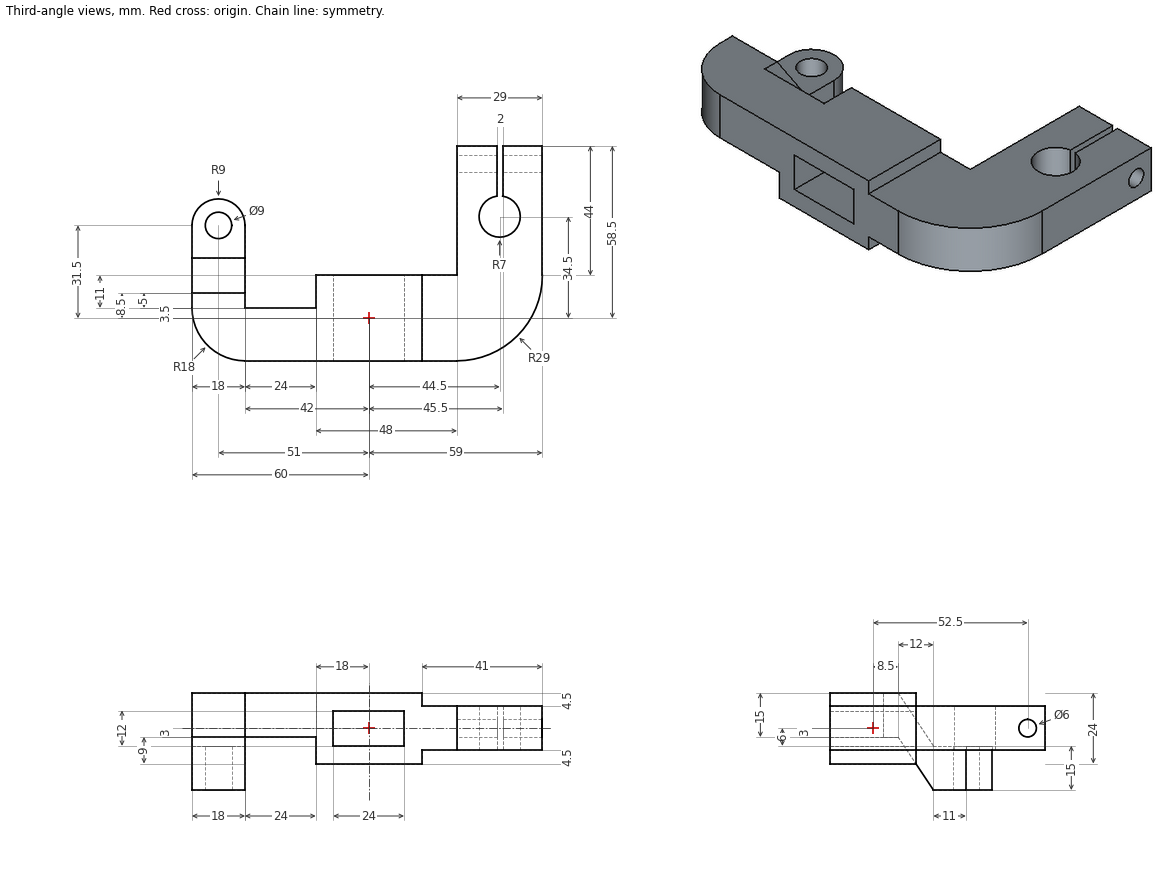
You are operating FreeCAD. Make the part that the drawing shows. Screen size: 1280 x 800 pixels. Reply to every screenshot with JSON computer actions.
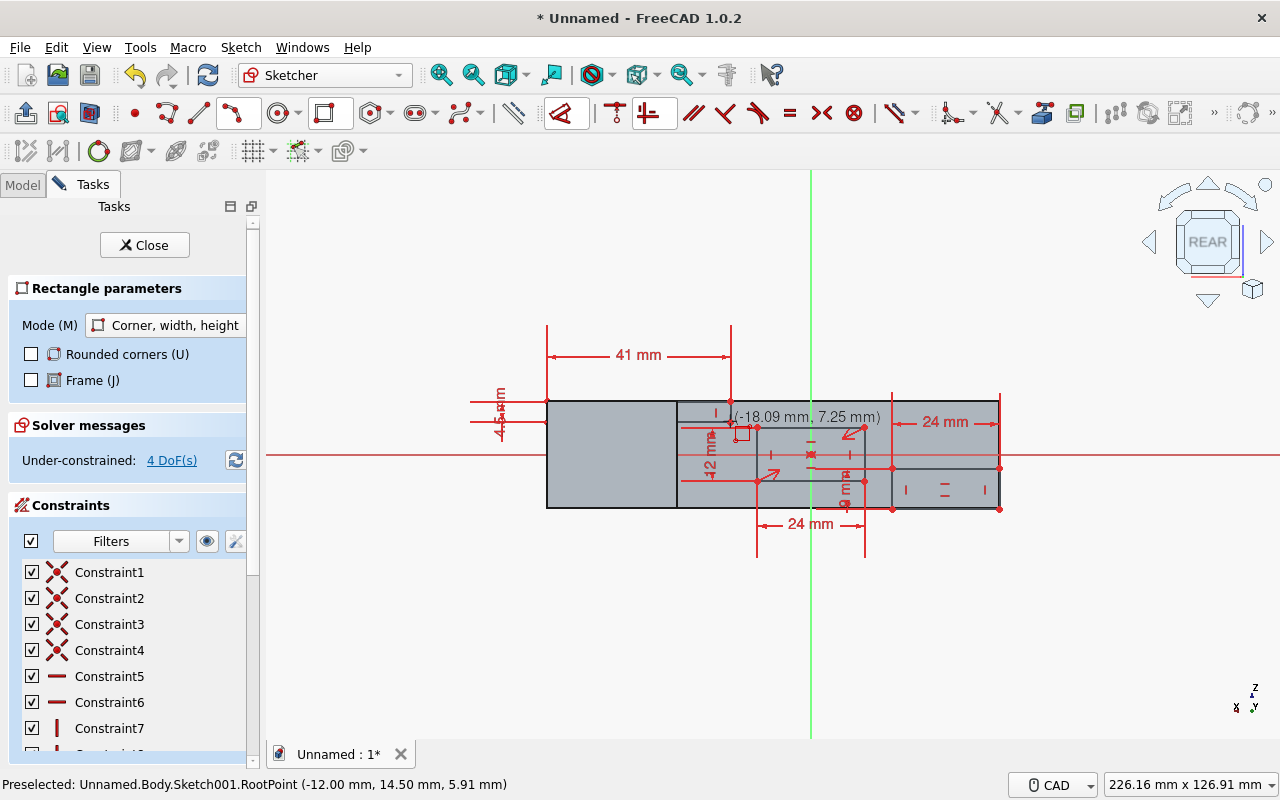
{"action": "left_click", "coordinate": [547, 488]}
{"action": "mouse_move", "coordinate": [730, 508]}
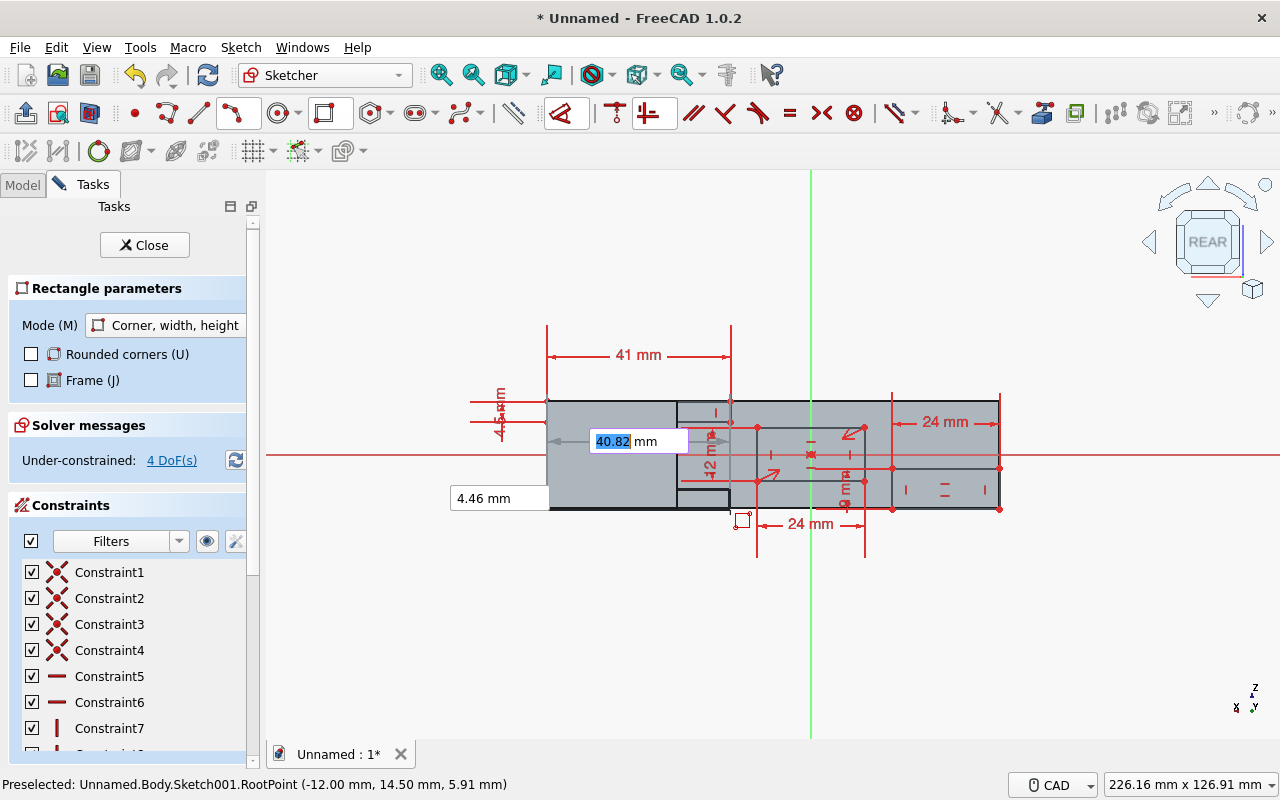
{"action": "type", "text": "41"}
{"action": "key", "text": "Tab"}
{"action": "type", "text": "4.5"}
{"action": "key", "text": "Return"}
{"action": "key", "text": "Escape"}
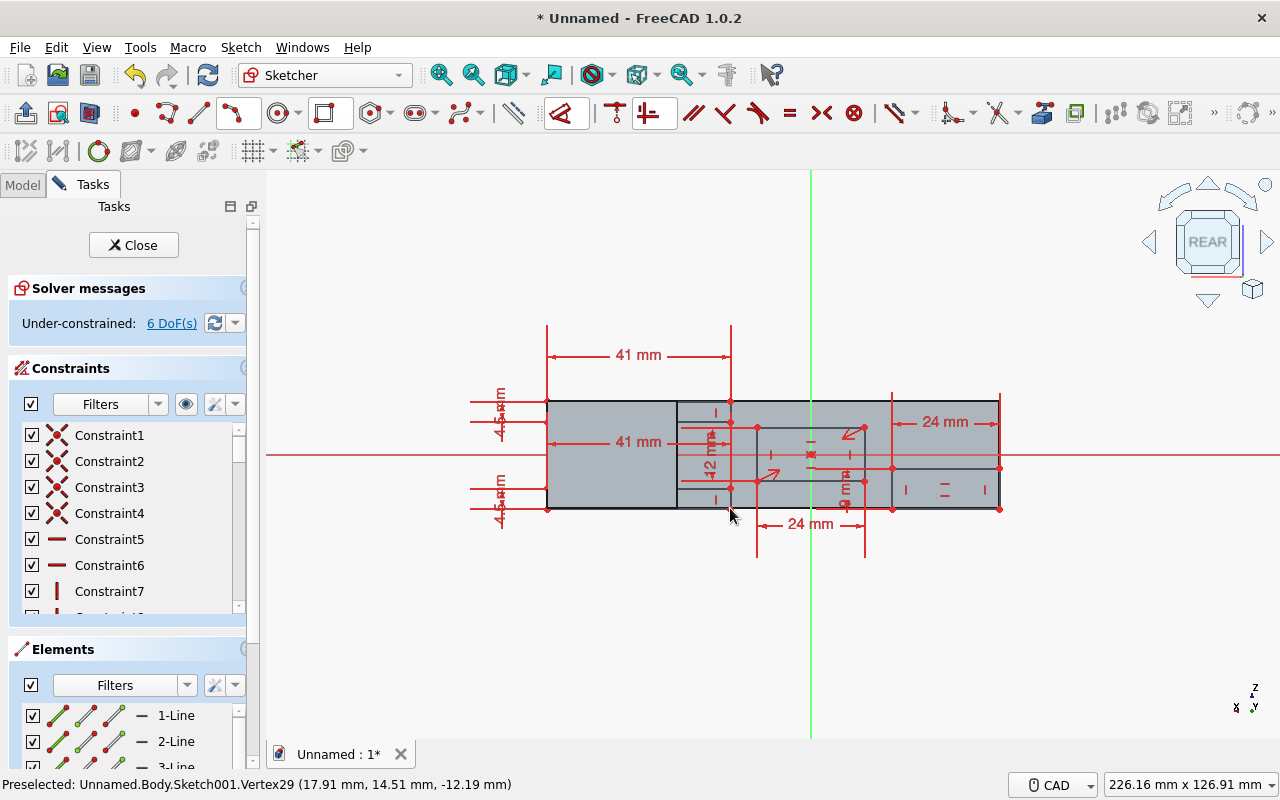
{"action": "left_click", "coordinate": [547, 422]}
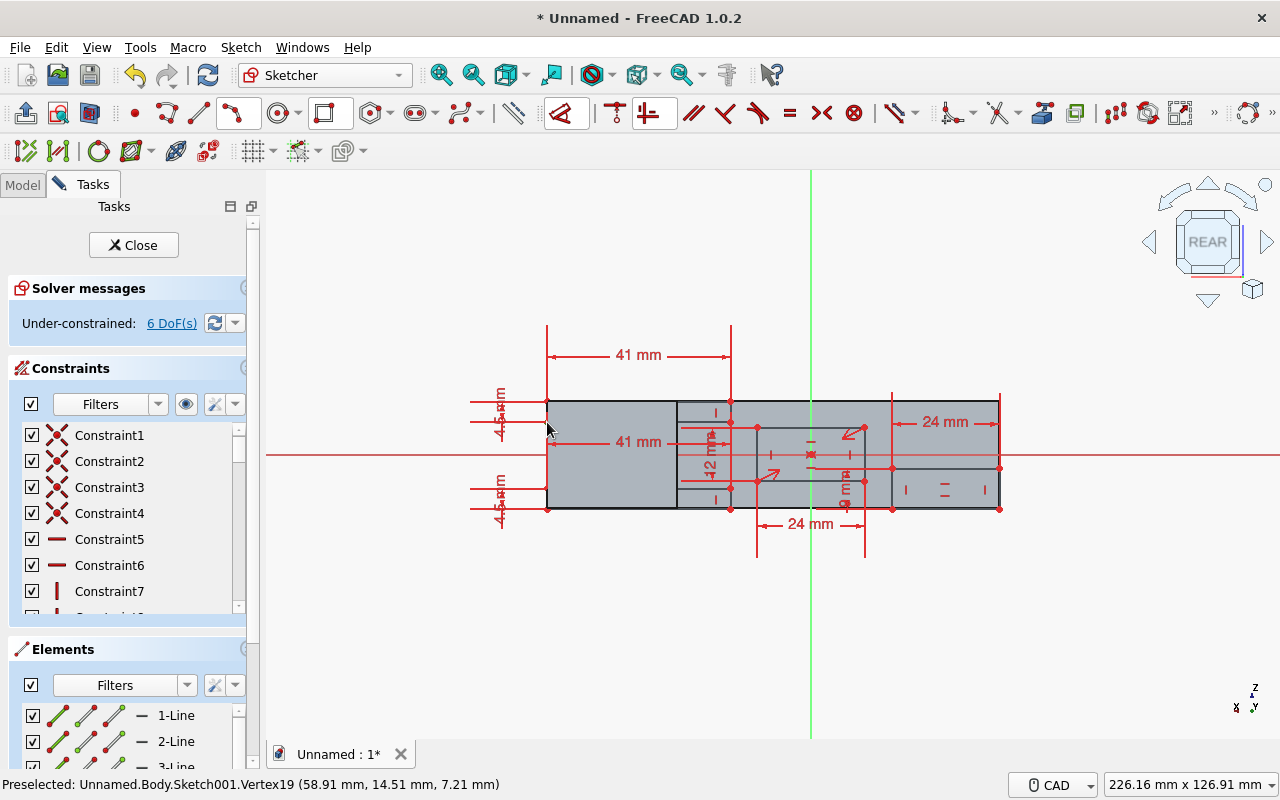
{"action": "left_click", "coordinate": [547, 489]}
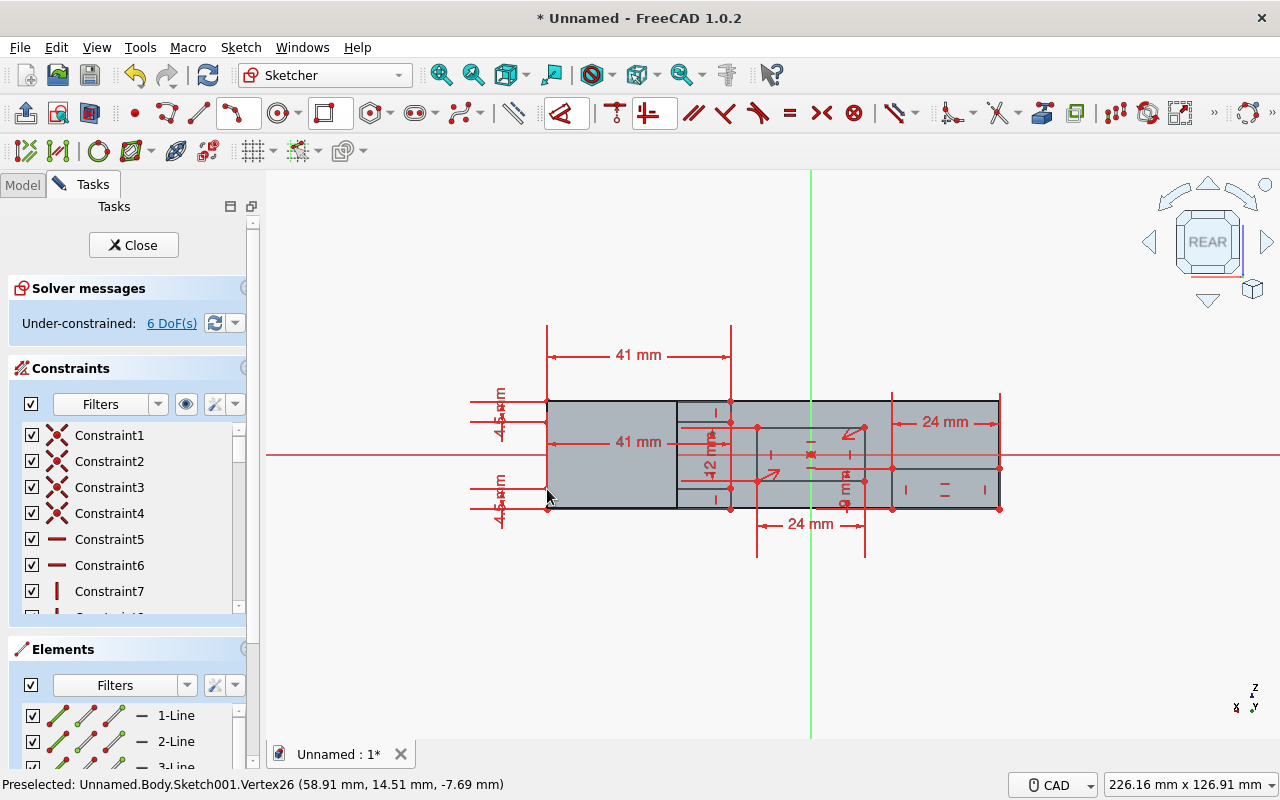
{"action": "left_click", "coordinate": [353, 454]}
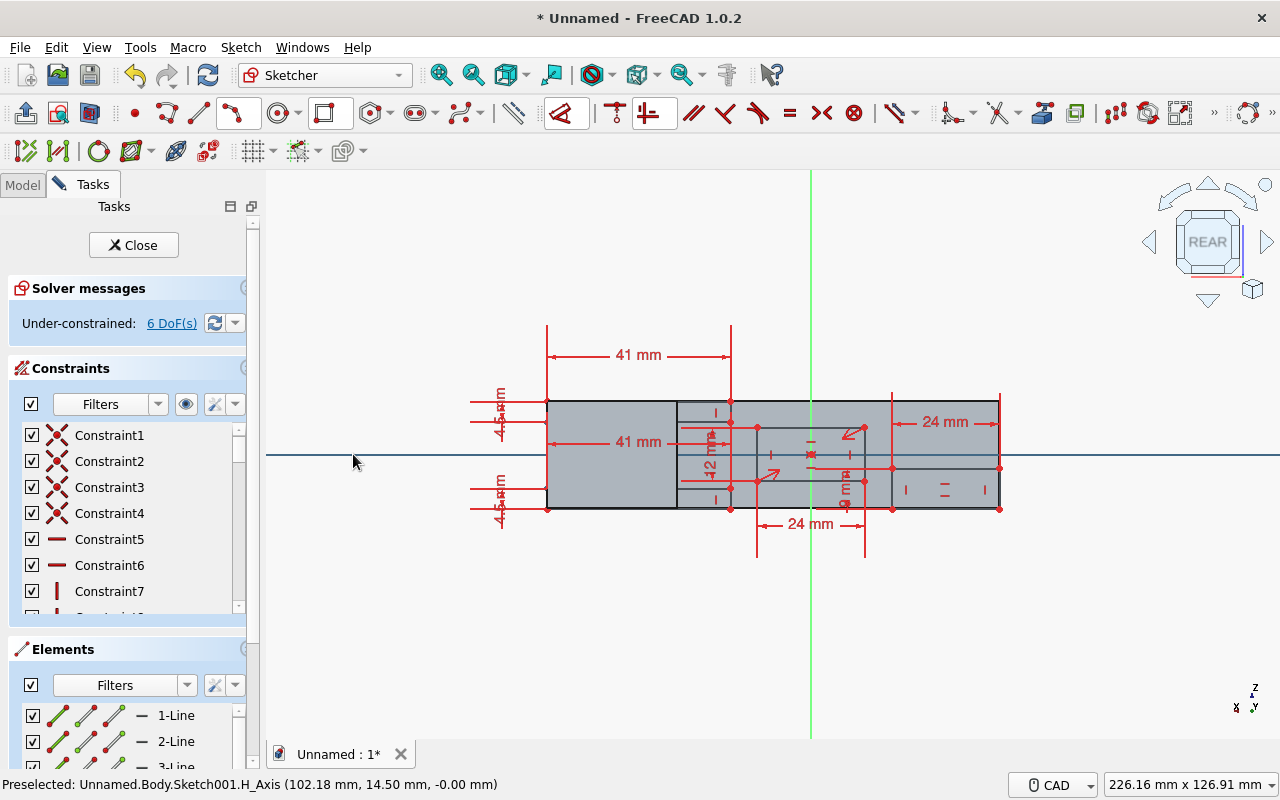
{"action": "left_click", "coordinate": [822, 114]}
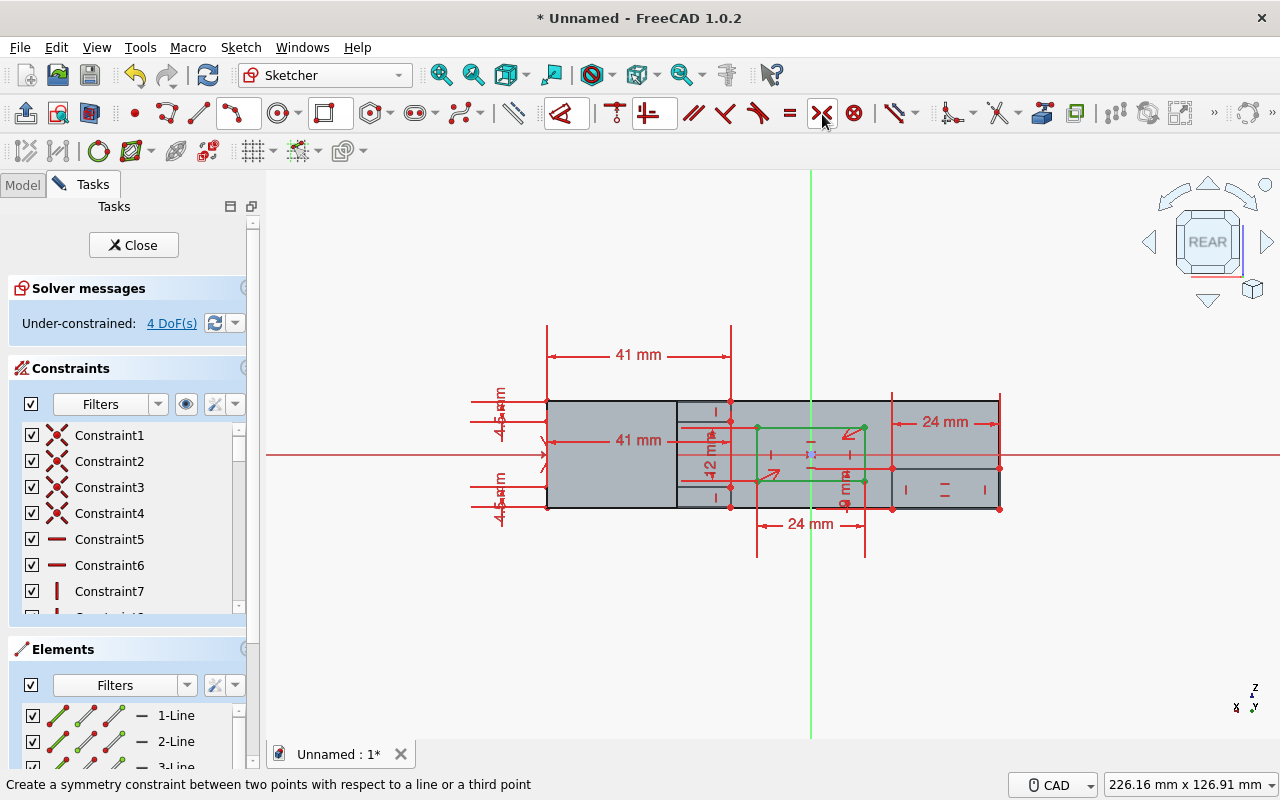
{"action": "left_click", "coordinate": [892, 509]}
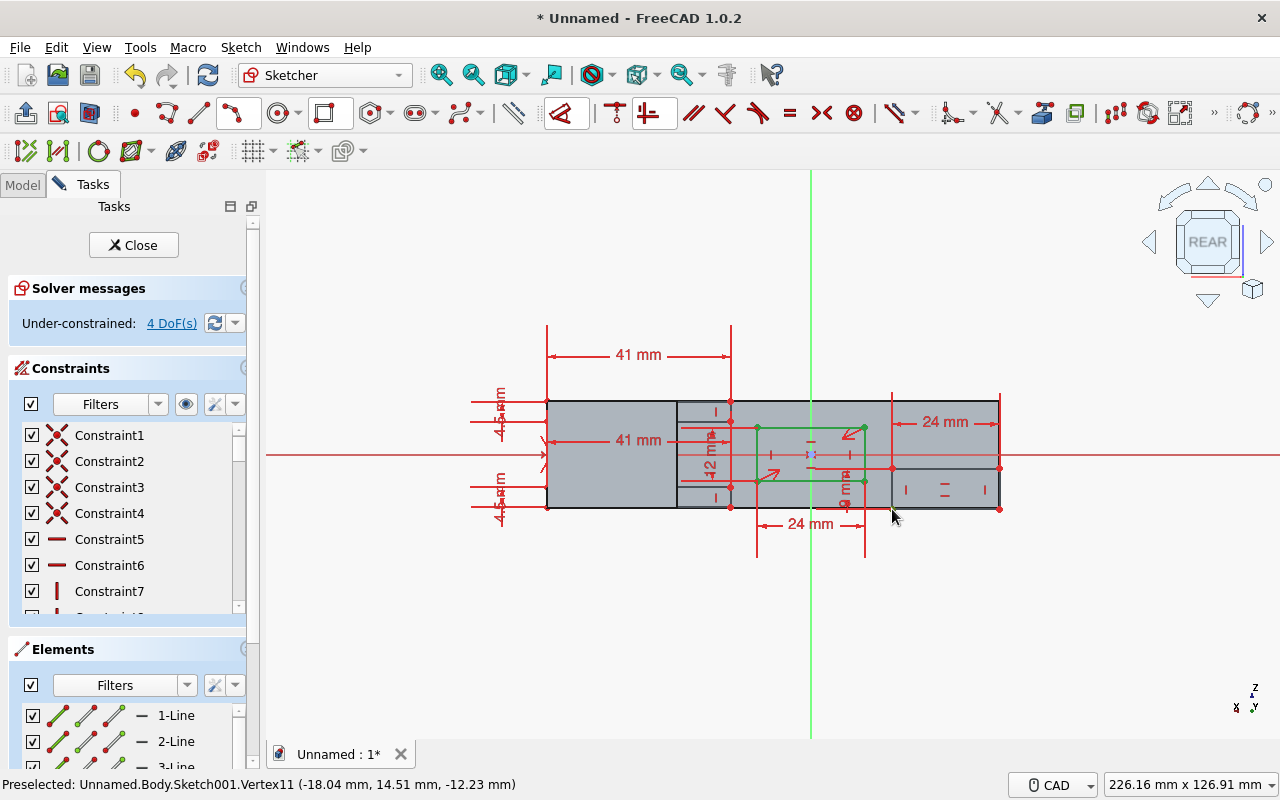
{"action": "left_click", "coordinate": [731, 507]}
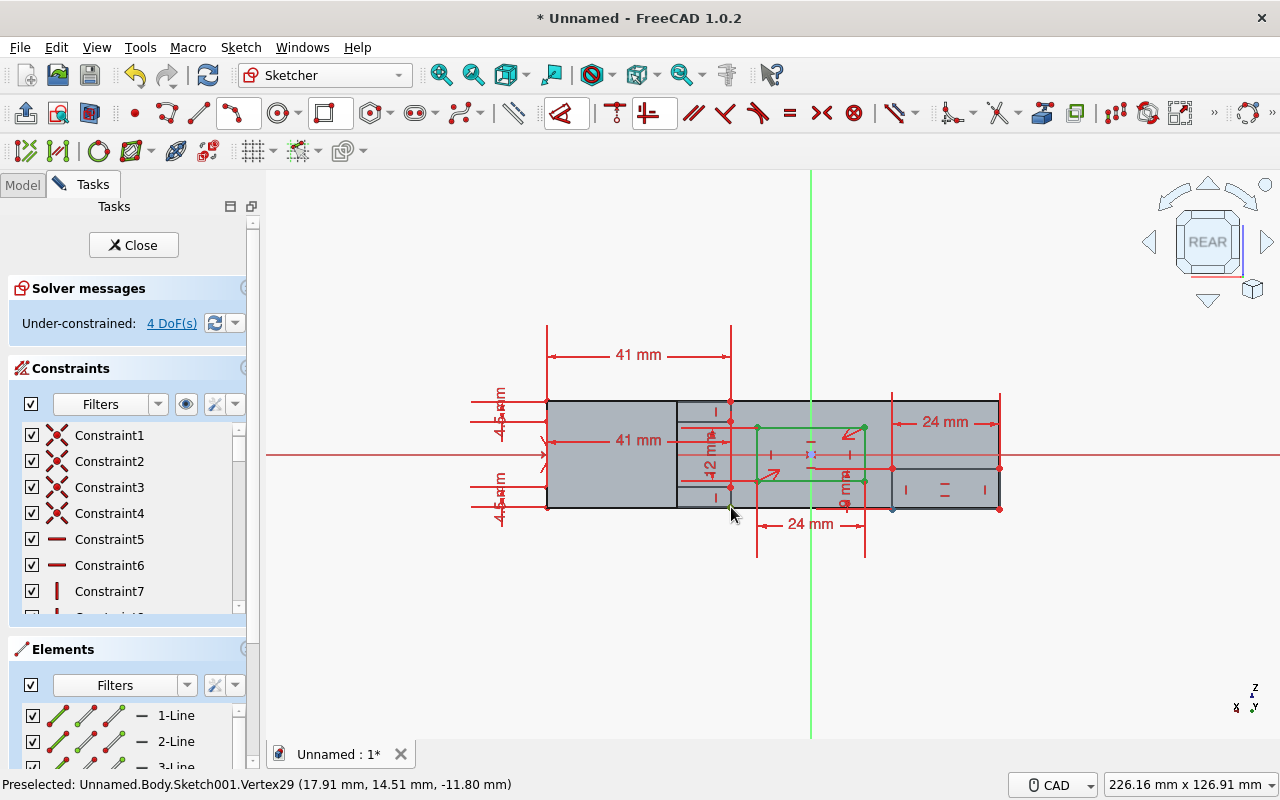
{"action": "left_click", "coordinate": [811, 674]}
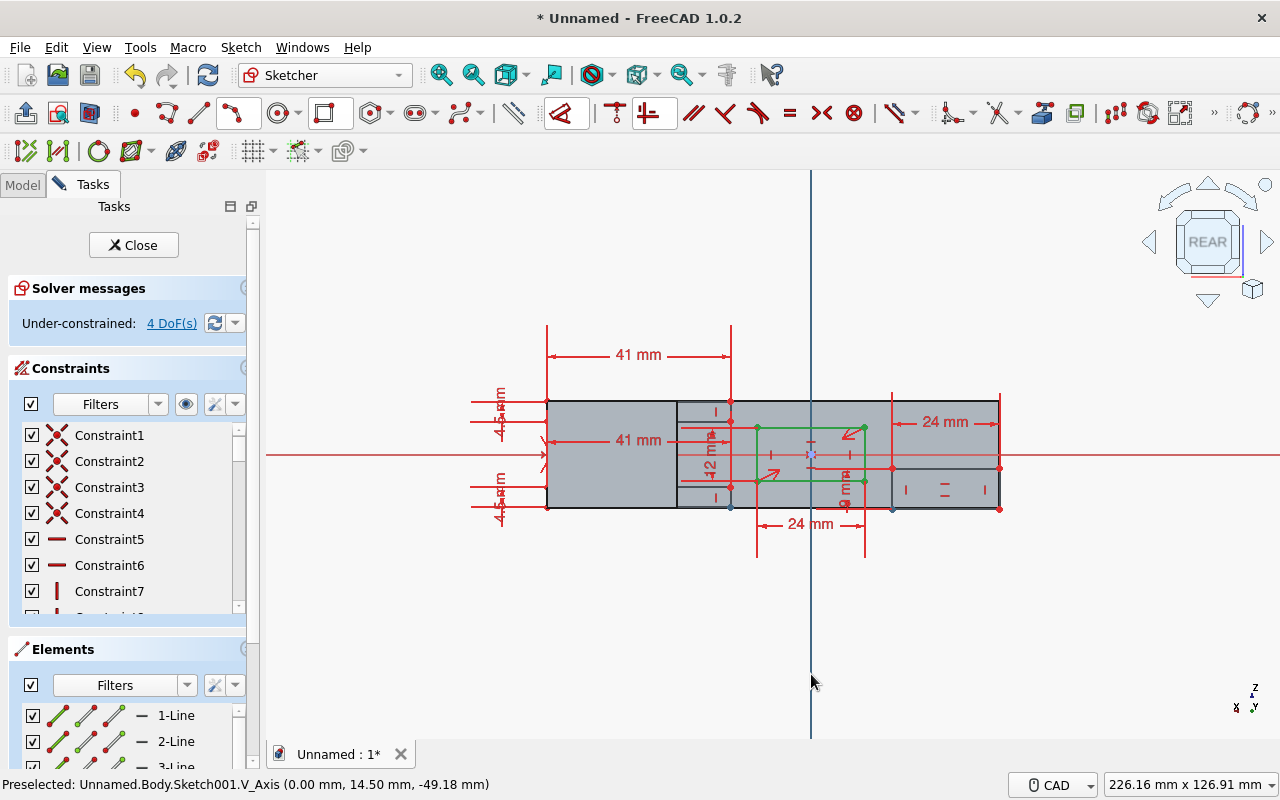
{"action": "left_click", "coordinate": [822, 114]}